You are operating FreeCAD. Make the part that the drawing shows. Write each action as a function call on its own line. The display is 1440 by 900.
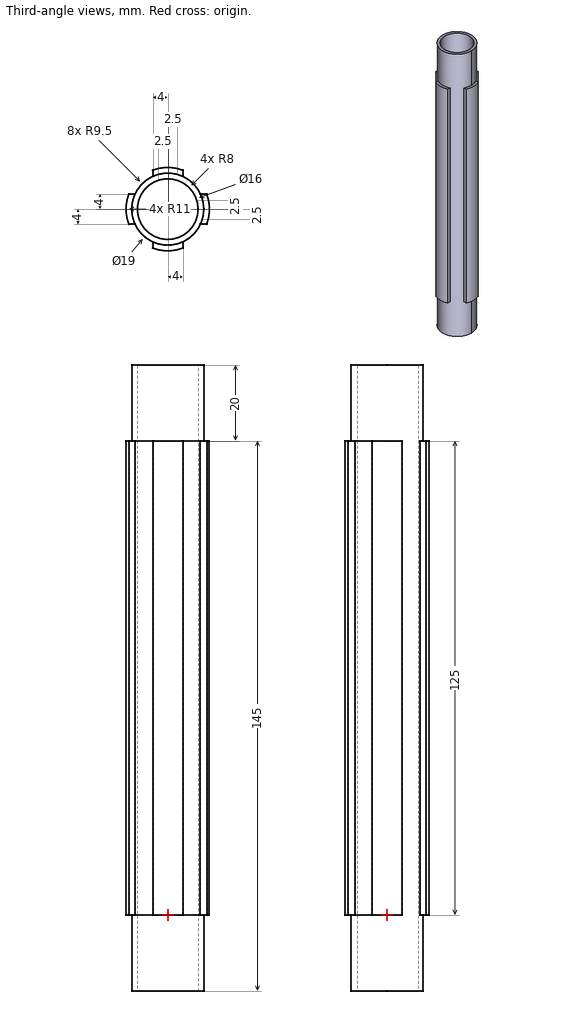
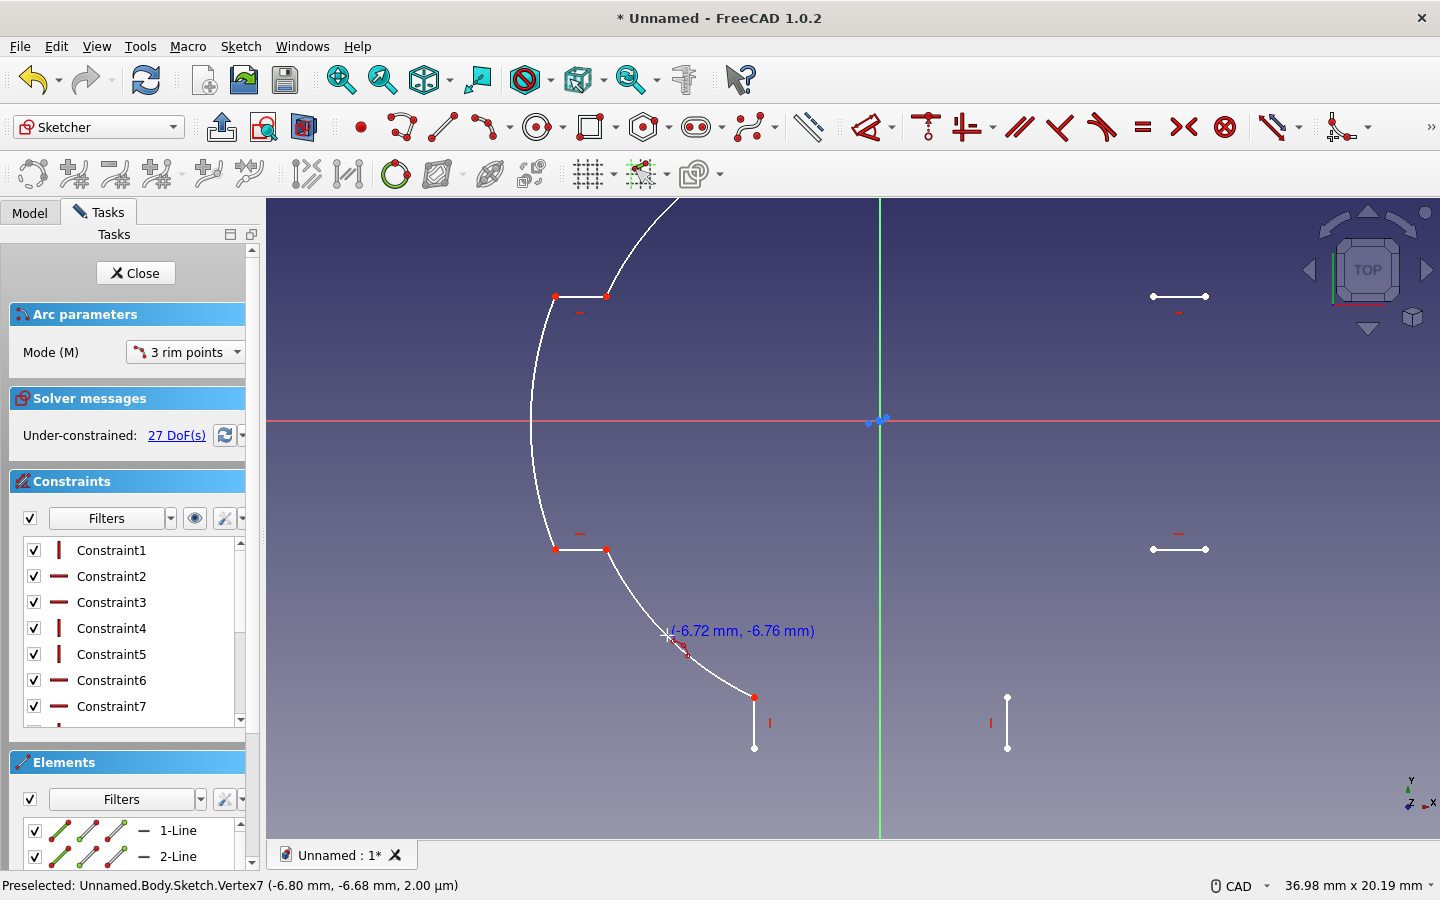
click(754, 748)
click(1007, 748)
click(854, 770)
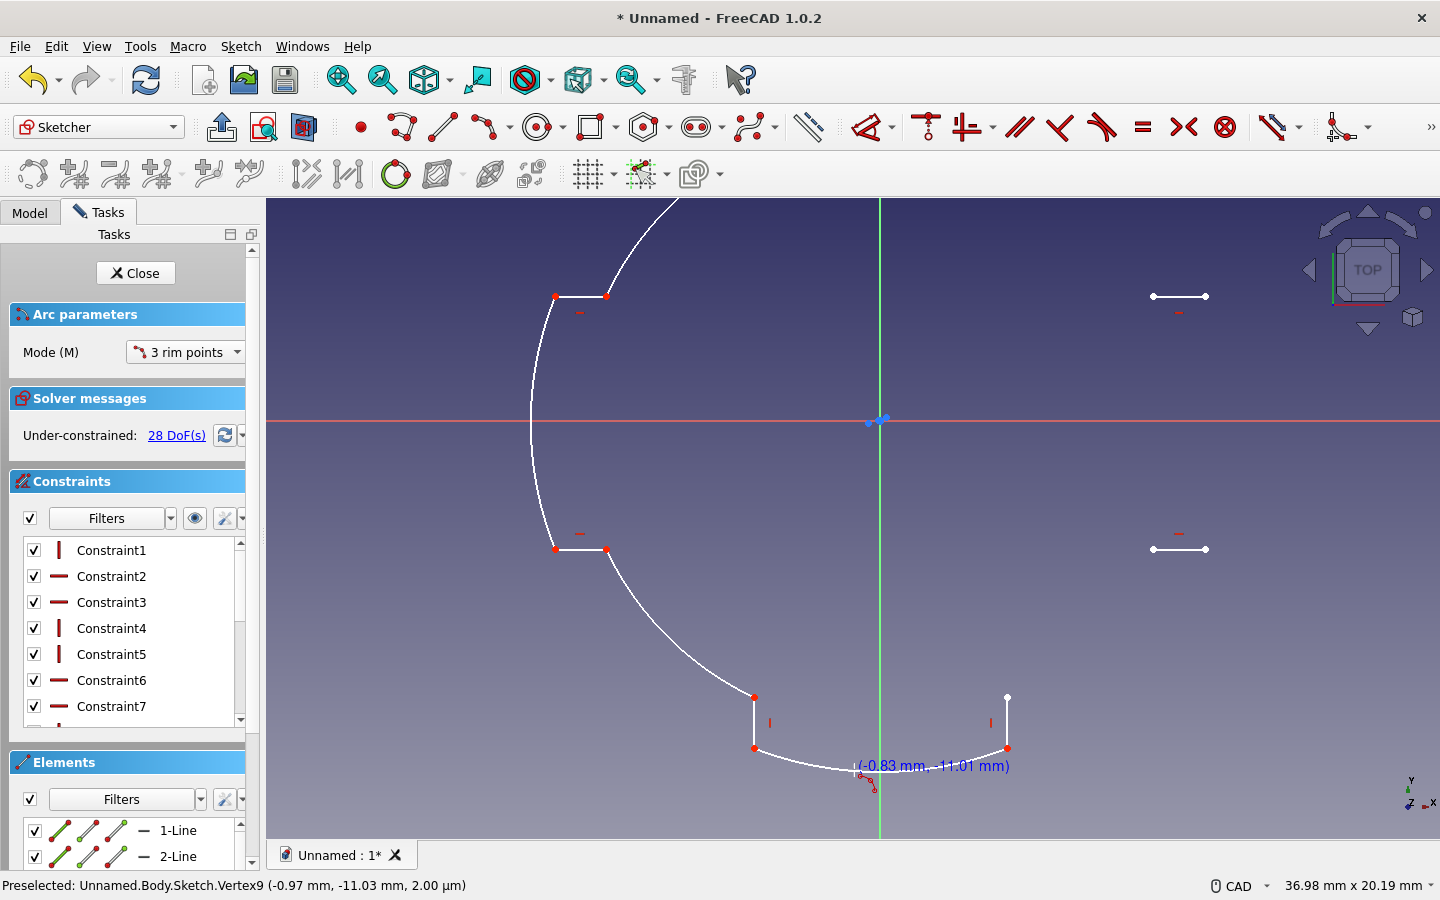
click(1007, 697)
click(1153, 550)
click(1094, 635)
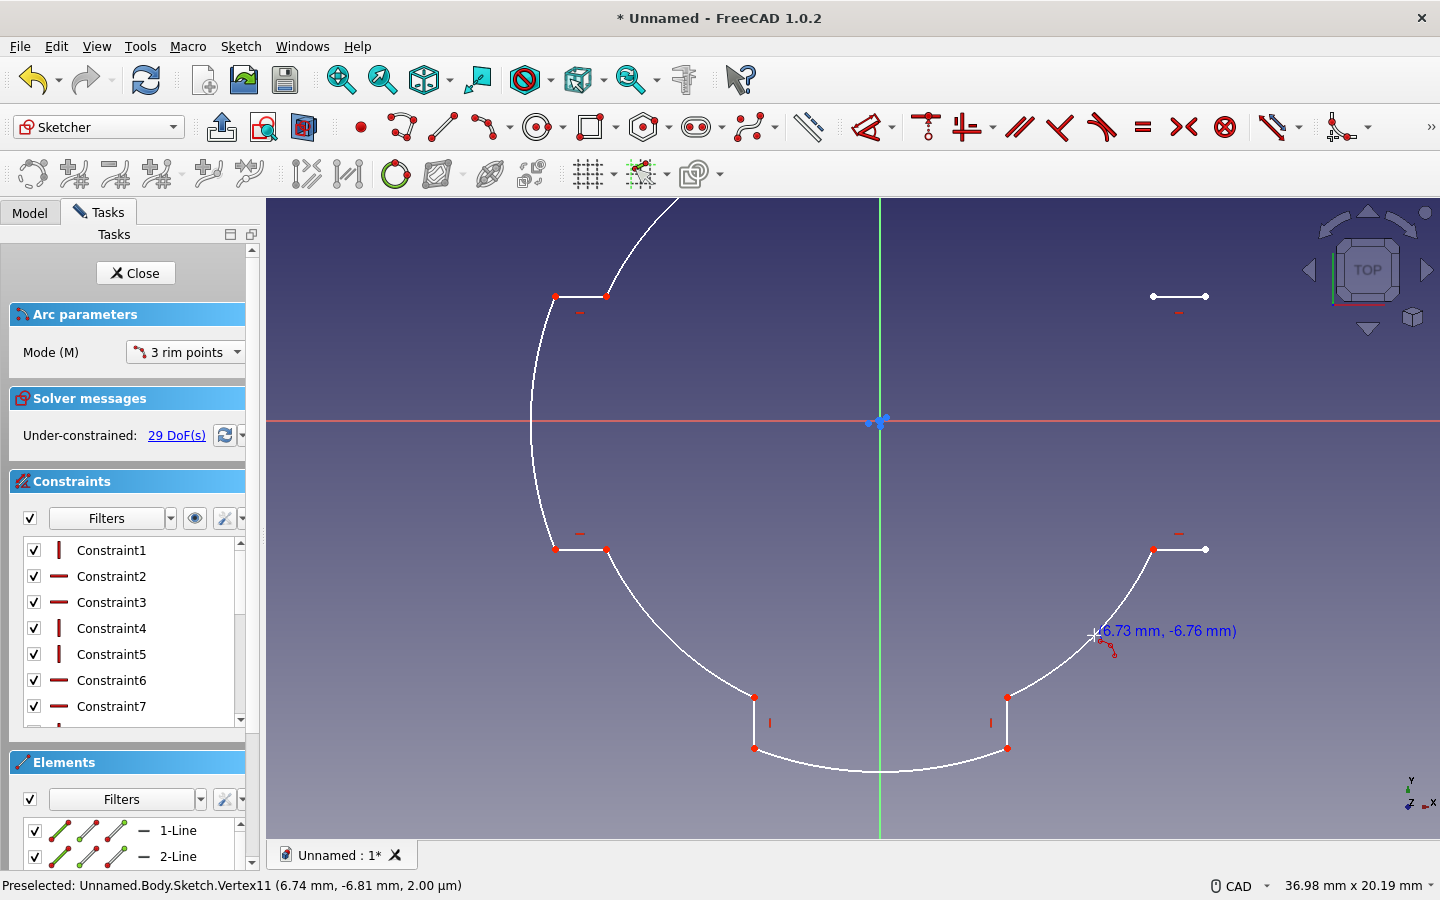
click(1206, 550)
click(1206, 297)
click(1229, 447)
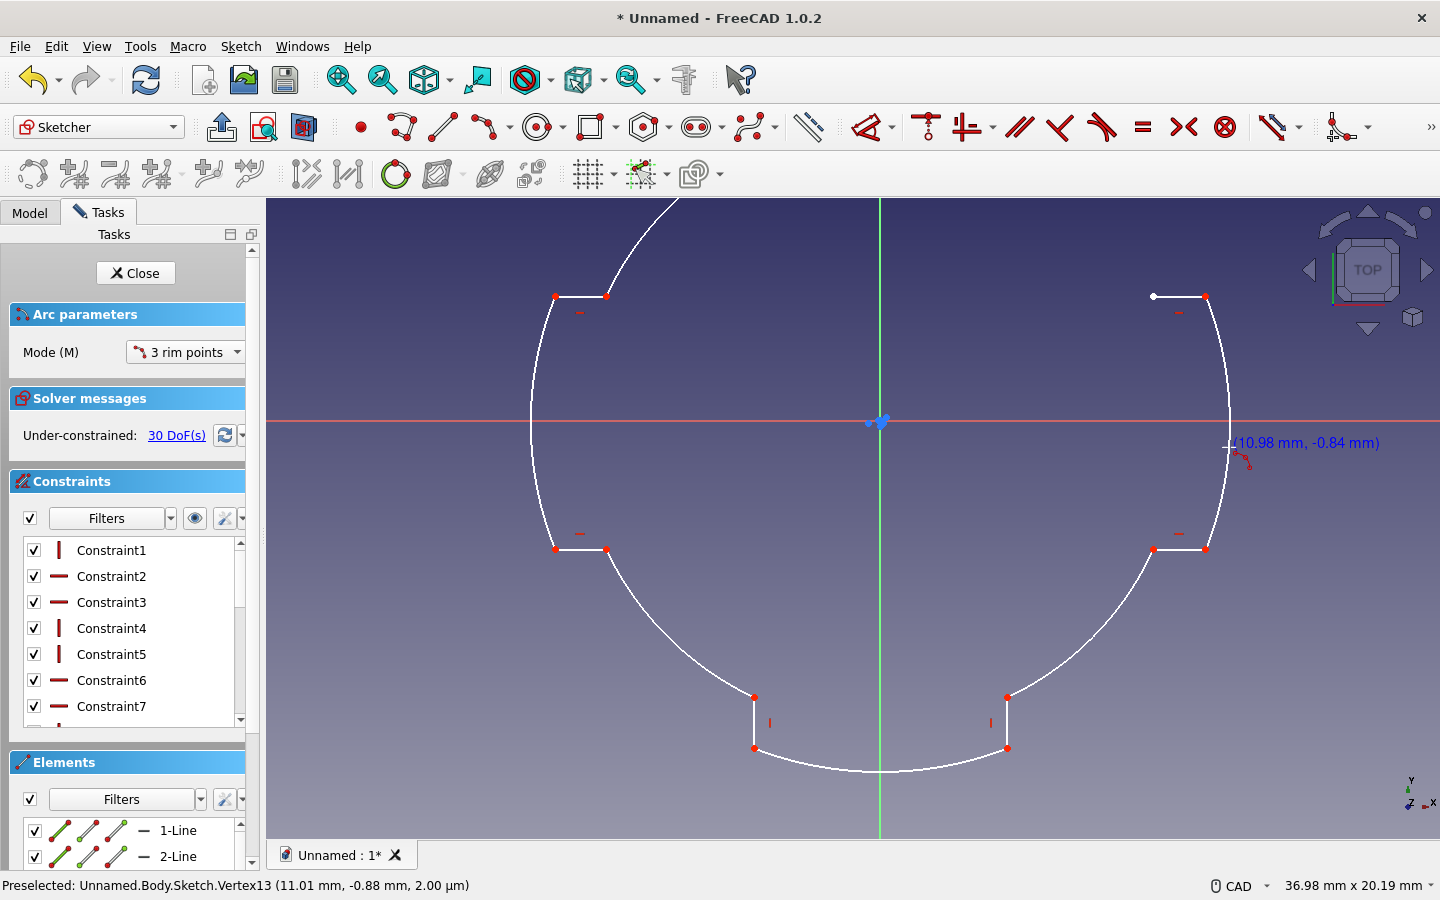
click(1153, 297)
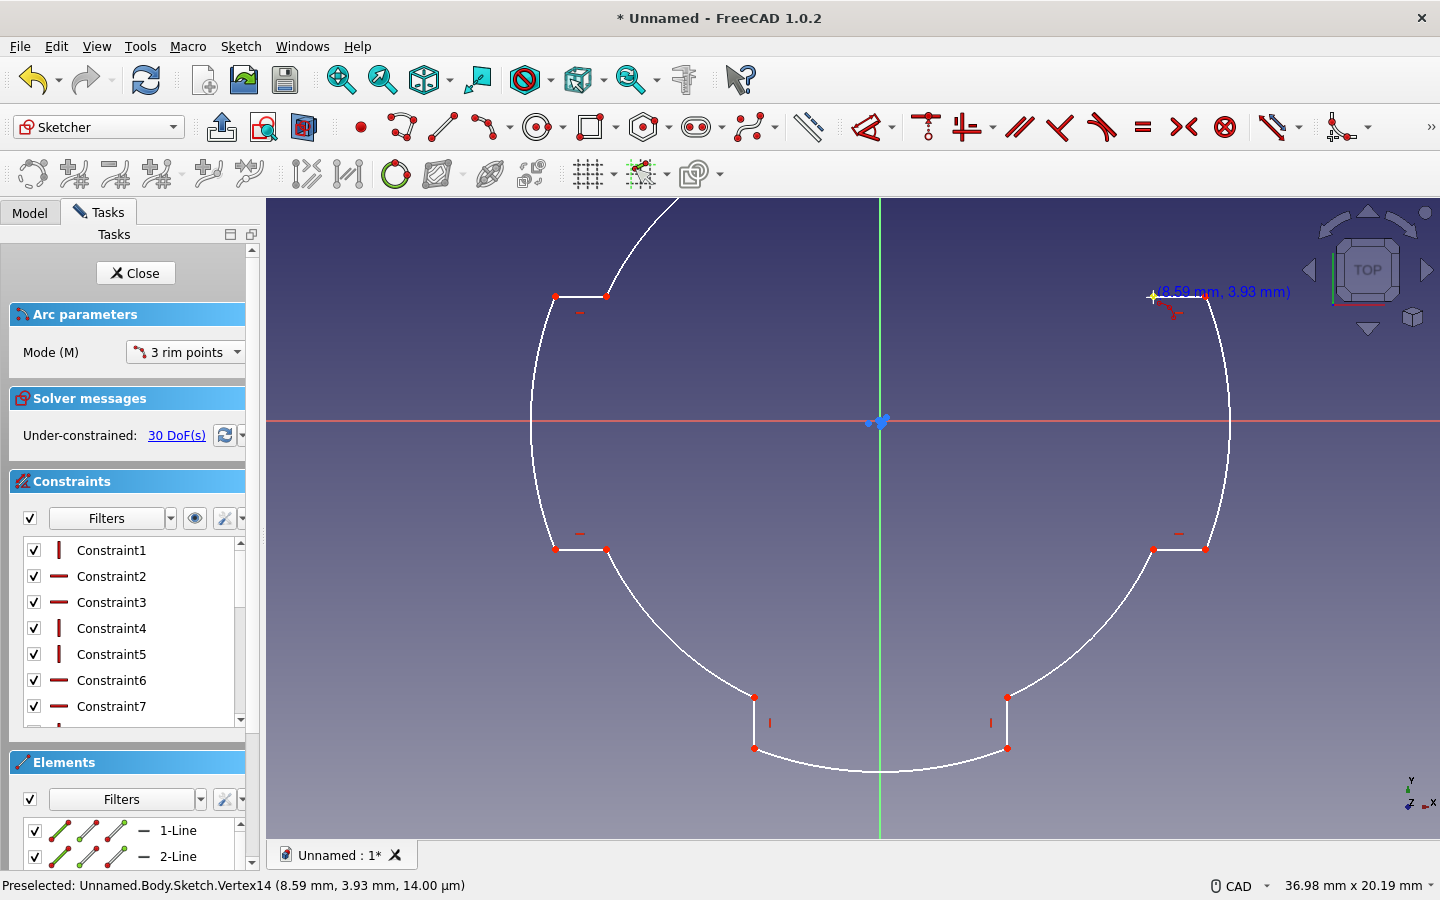
scroll(668, 637, down, 3)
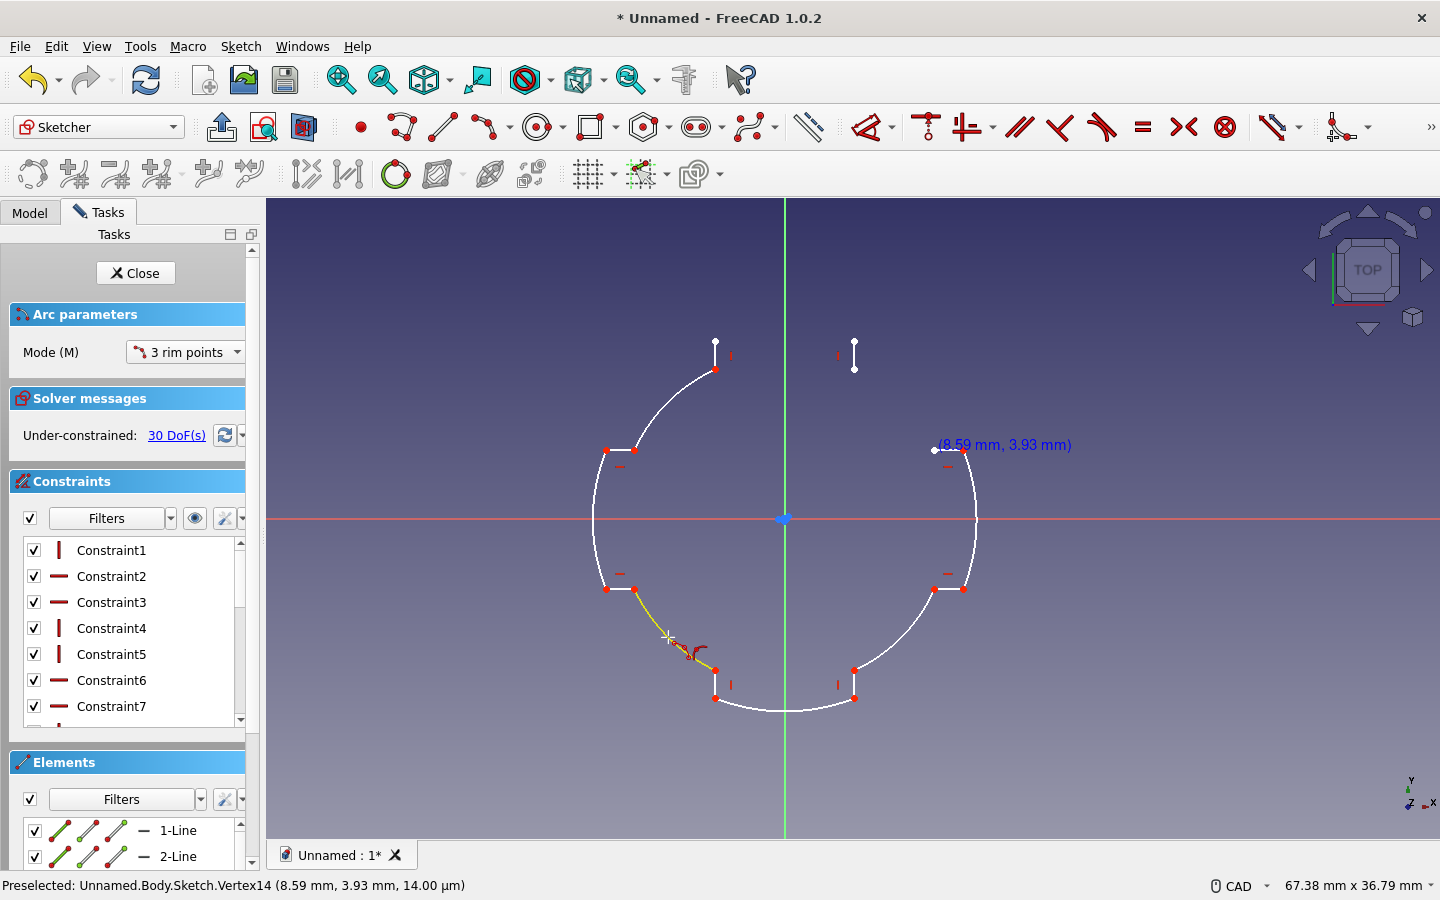
click(854, 369)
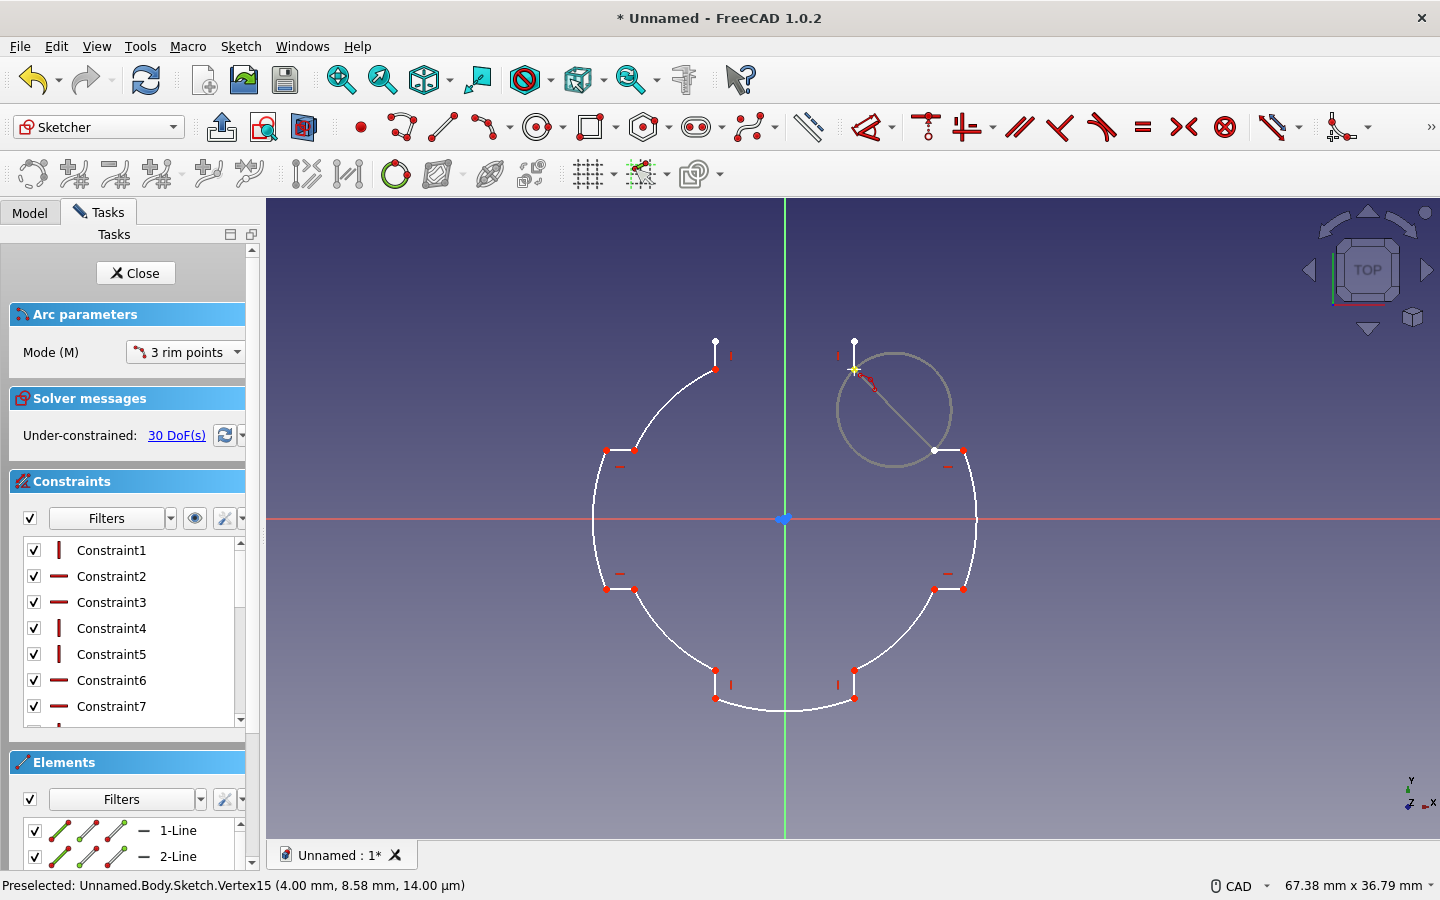
scroll(902, 402, up, 3)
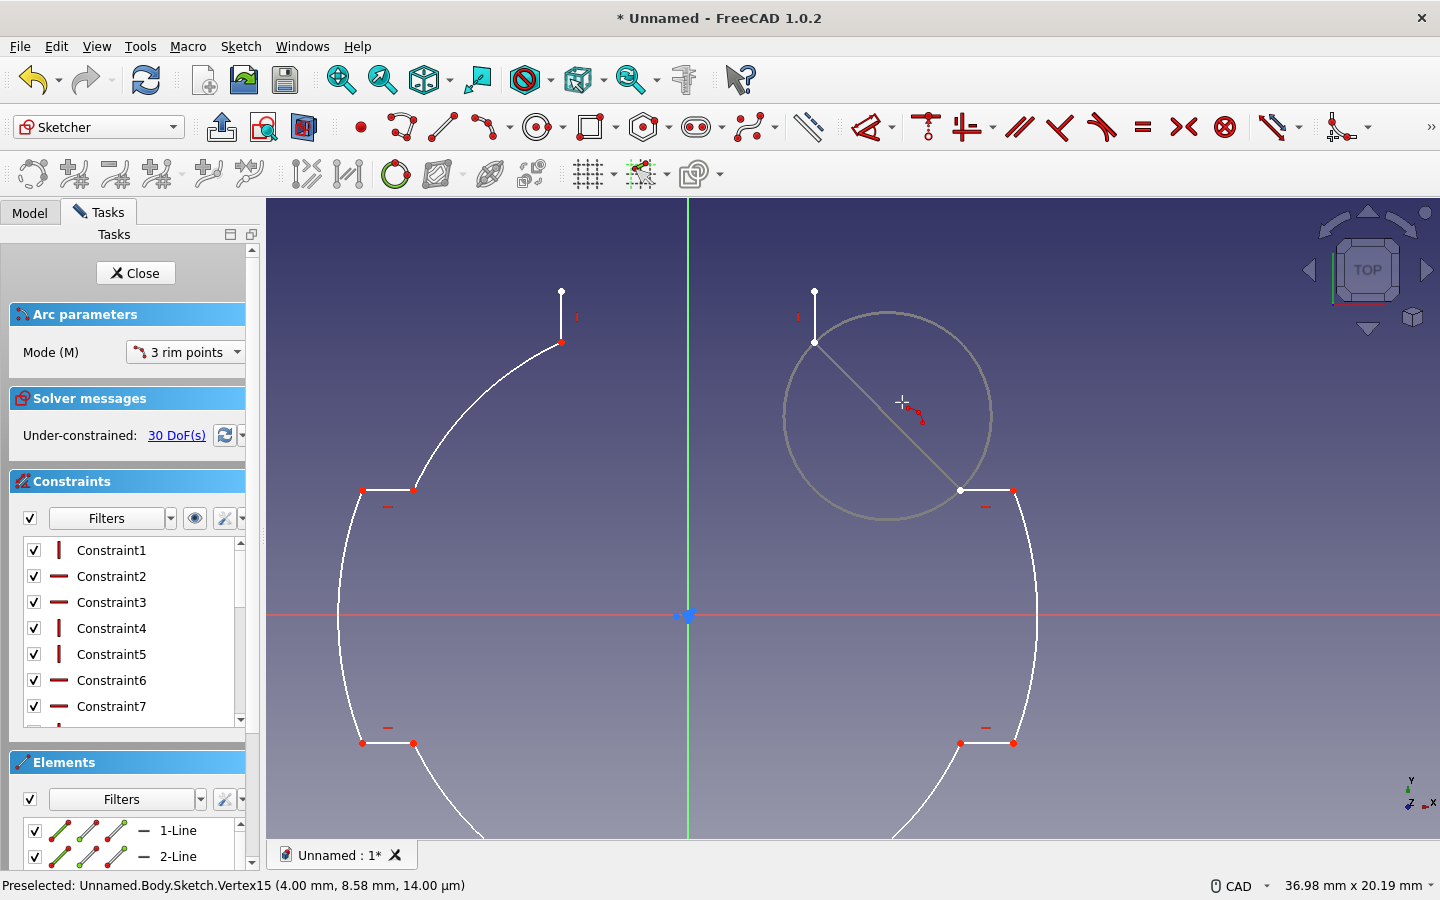
click(901, 402)